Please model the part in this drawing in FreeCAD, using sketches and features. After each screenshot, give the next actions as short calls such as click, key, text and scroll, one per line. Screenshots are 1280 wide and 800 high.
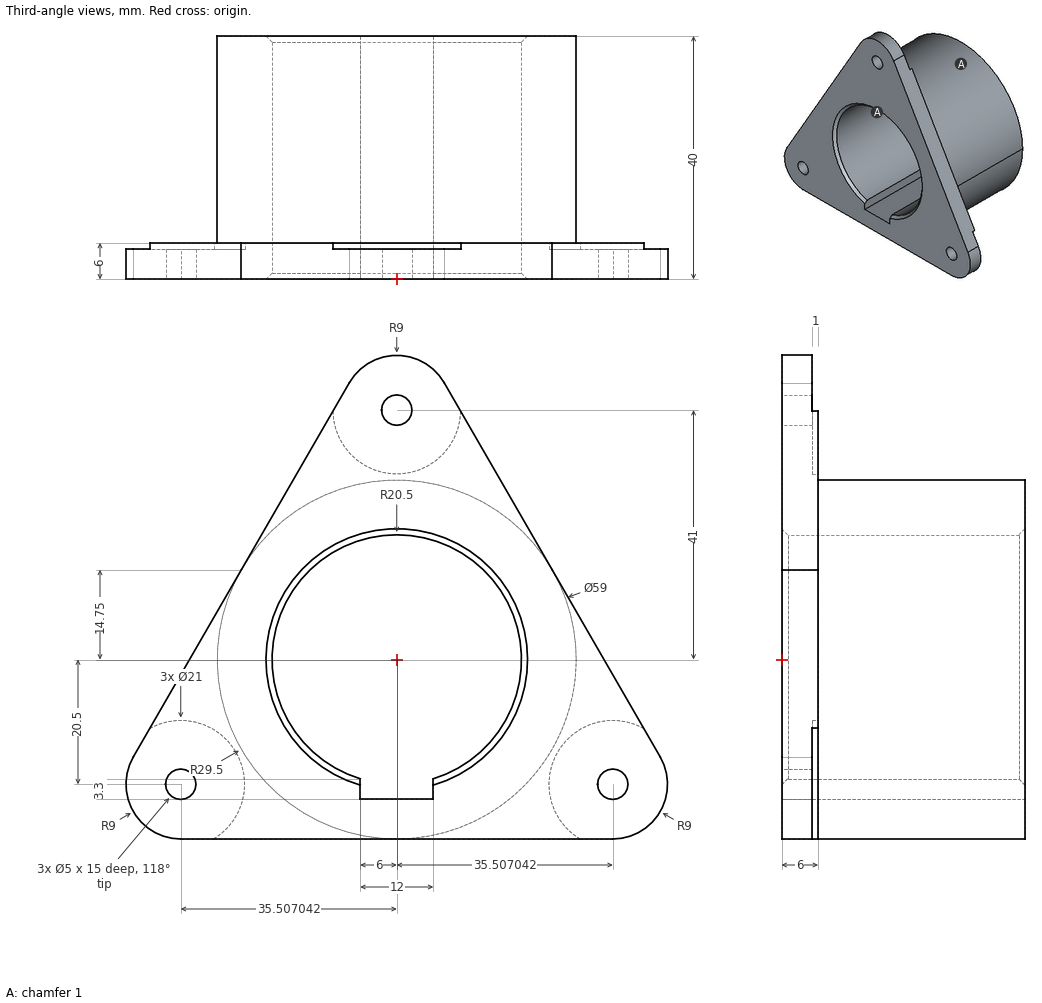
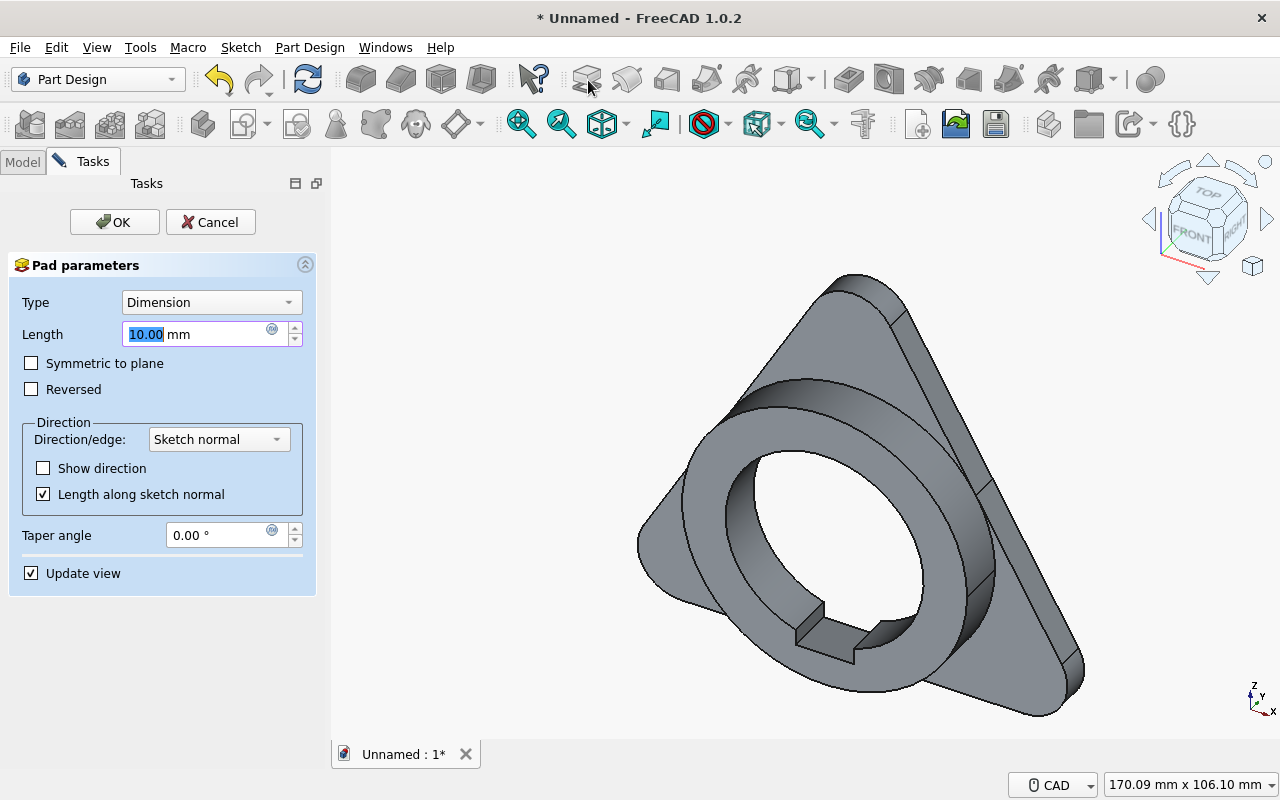
text(40)
key(Tab)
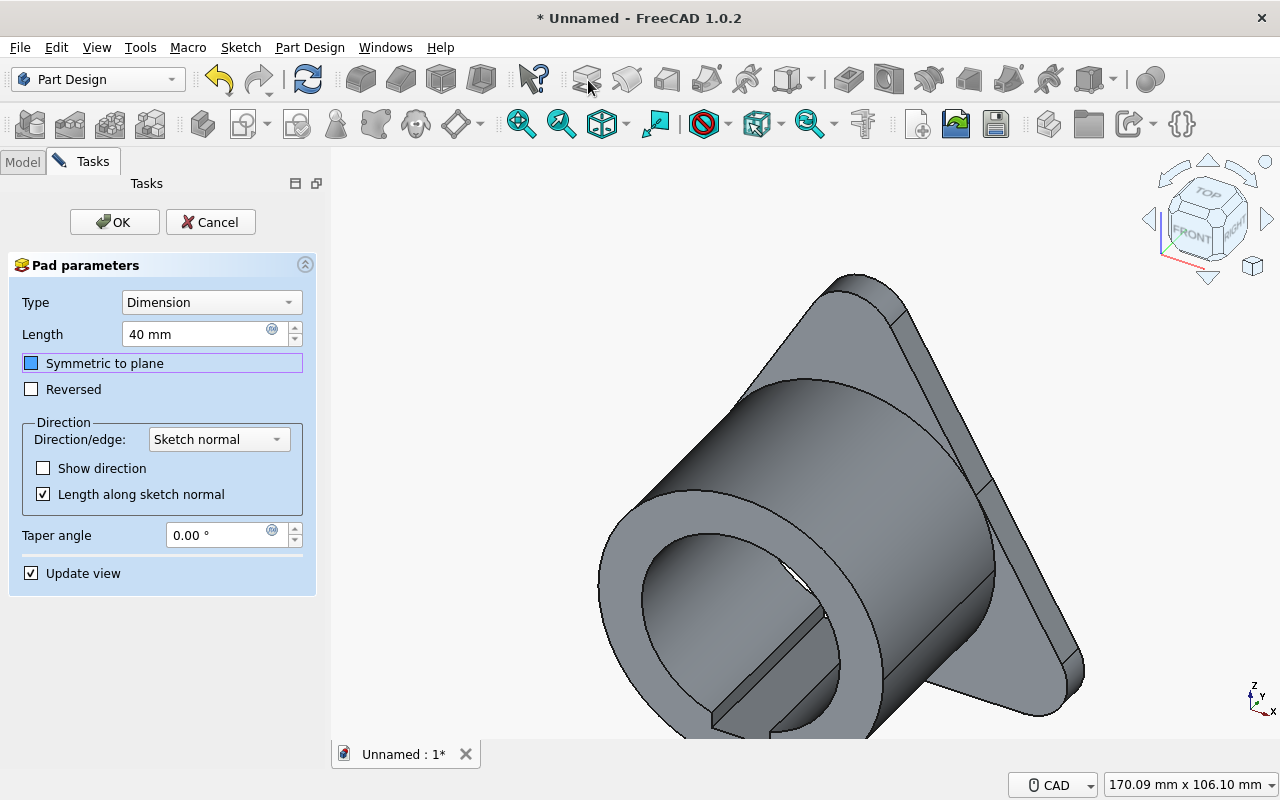
click(30, 389)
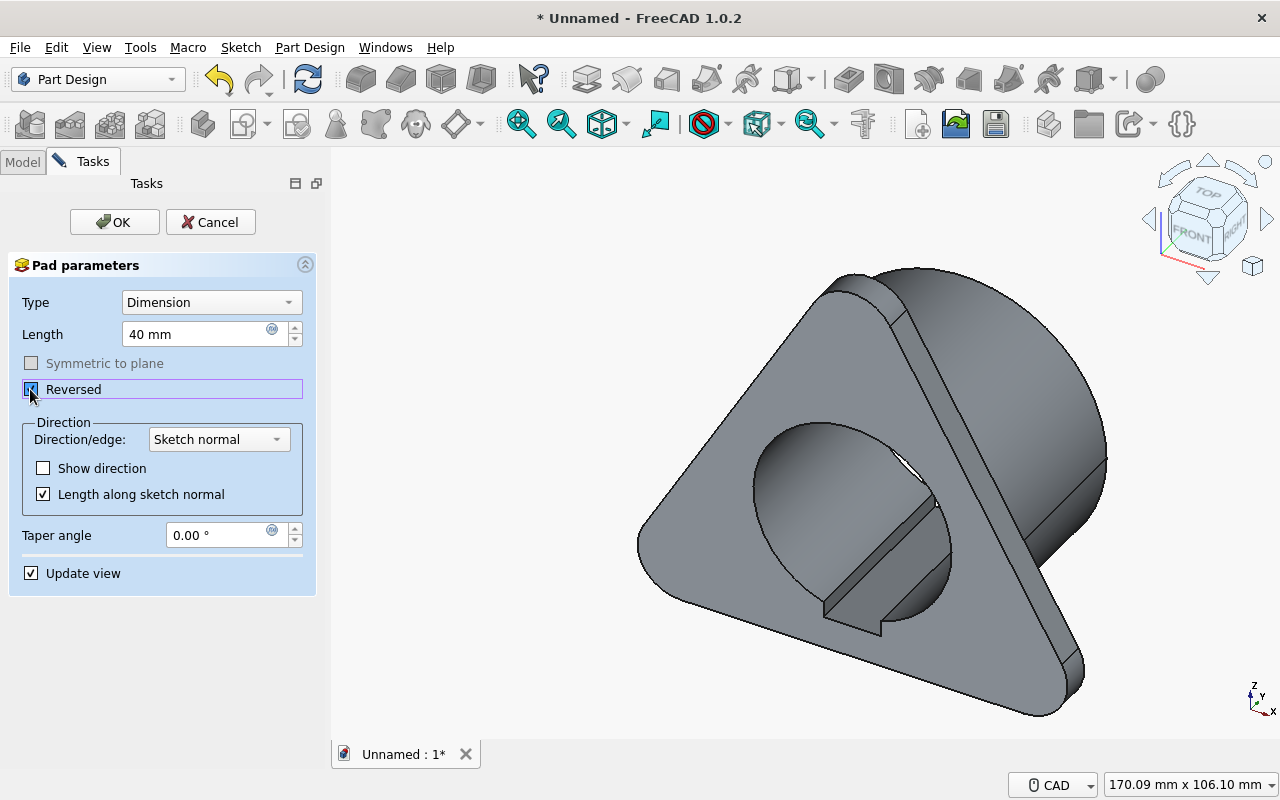
click(115, 222)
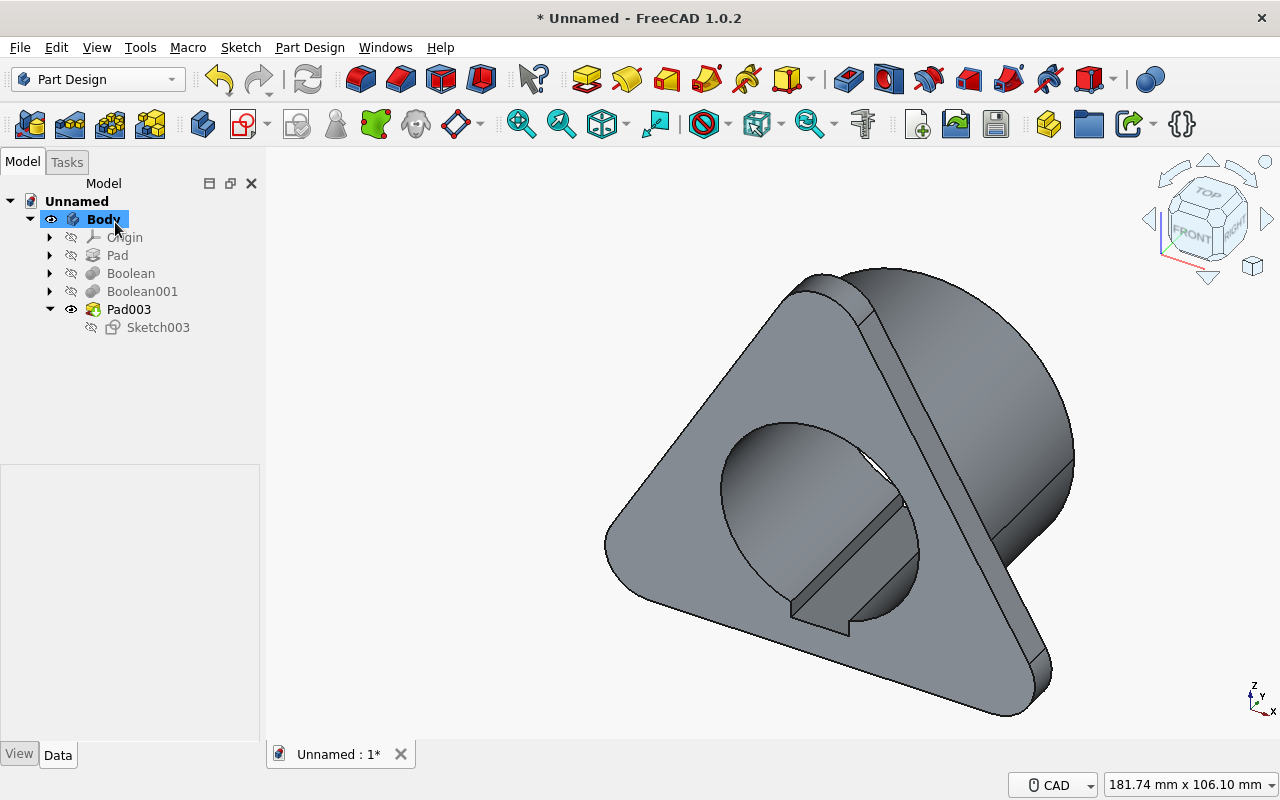
click(522, 124)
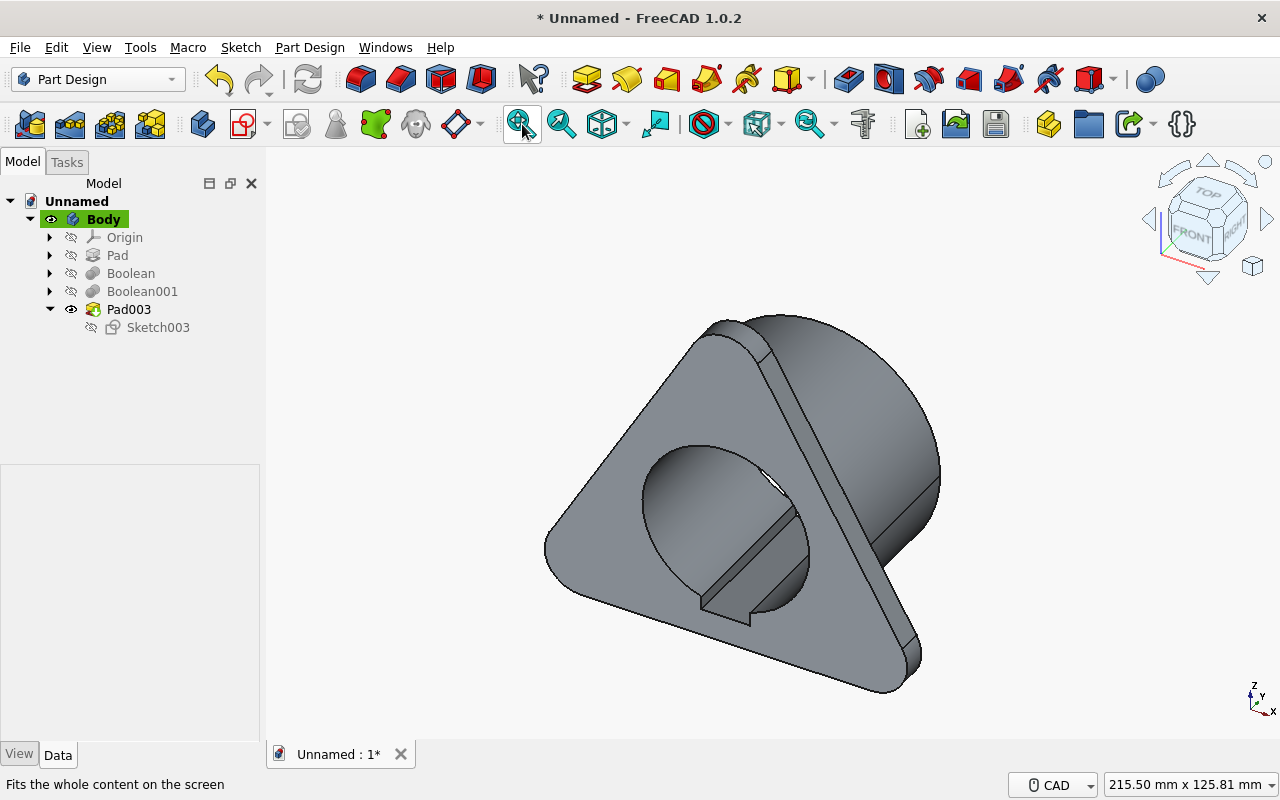
click(650, 470)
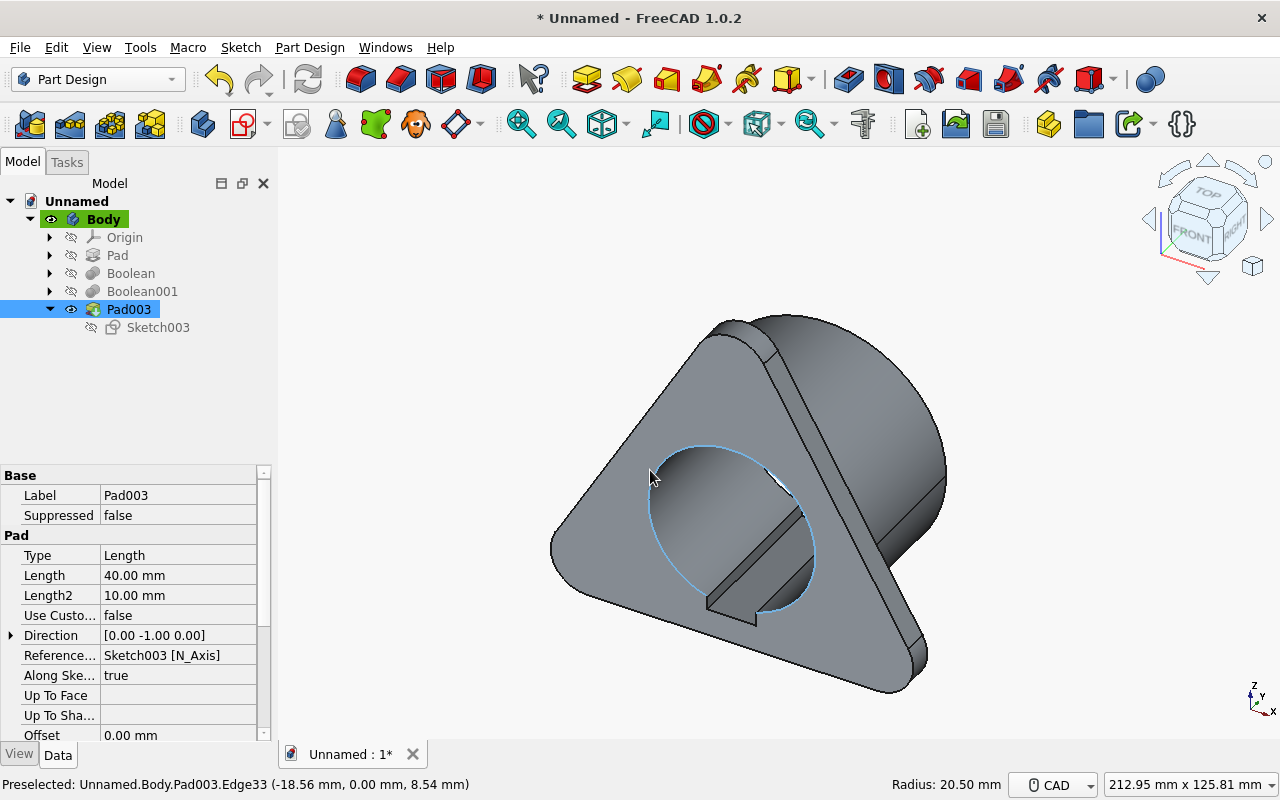
key(0)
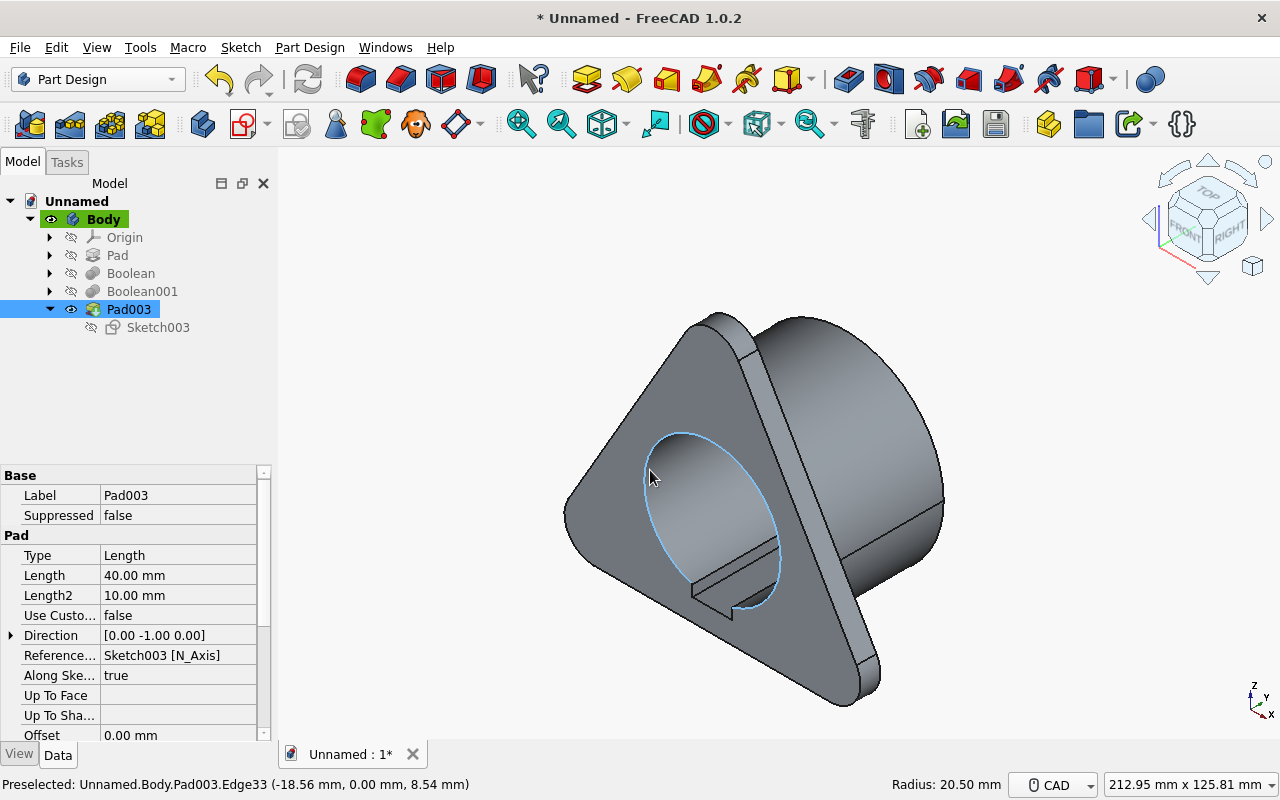
key(2)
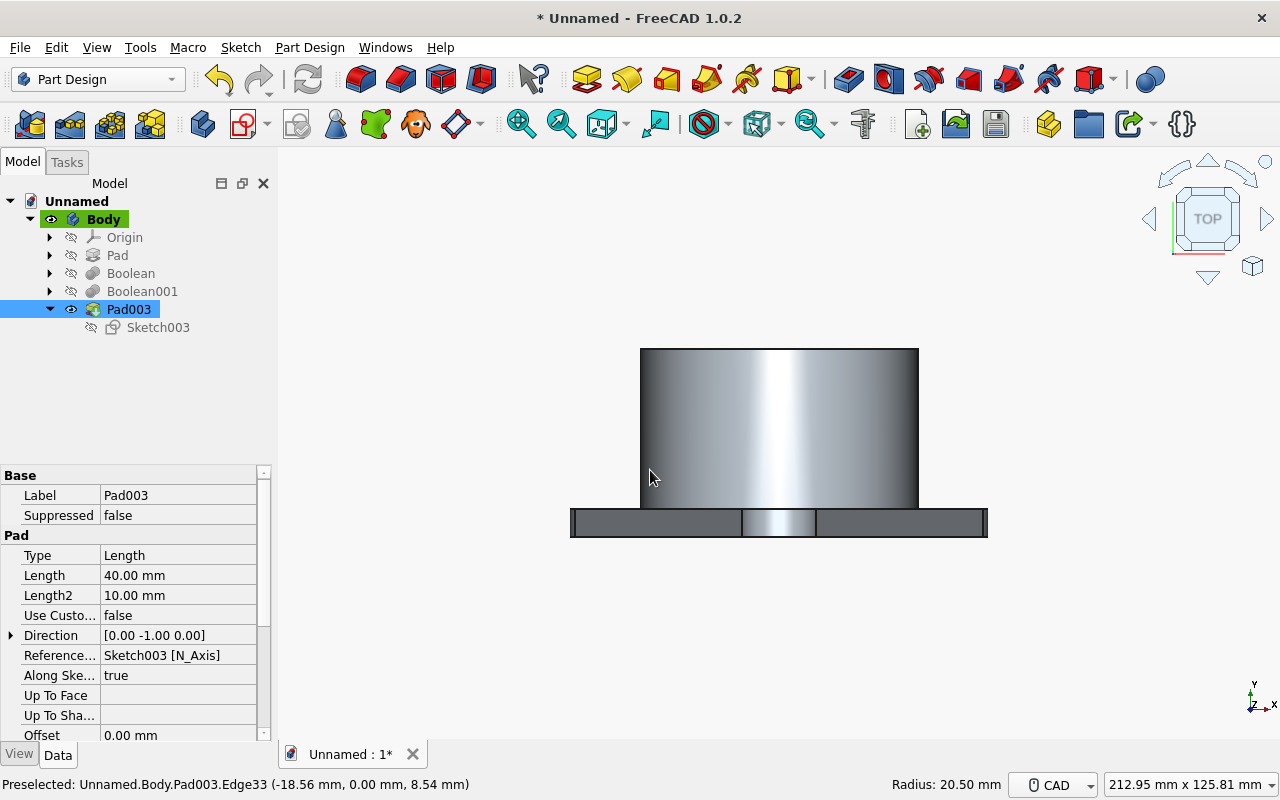
click(522, 124)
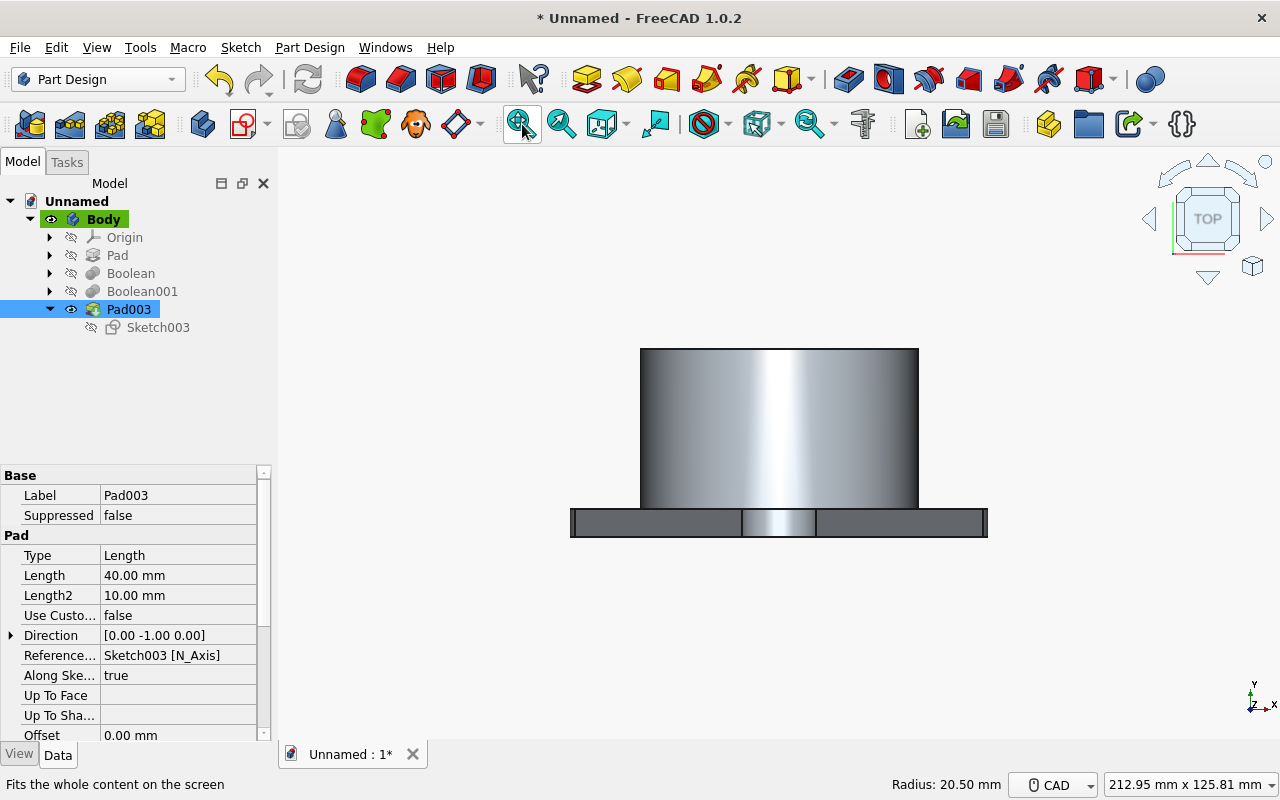
key(1)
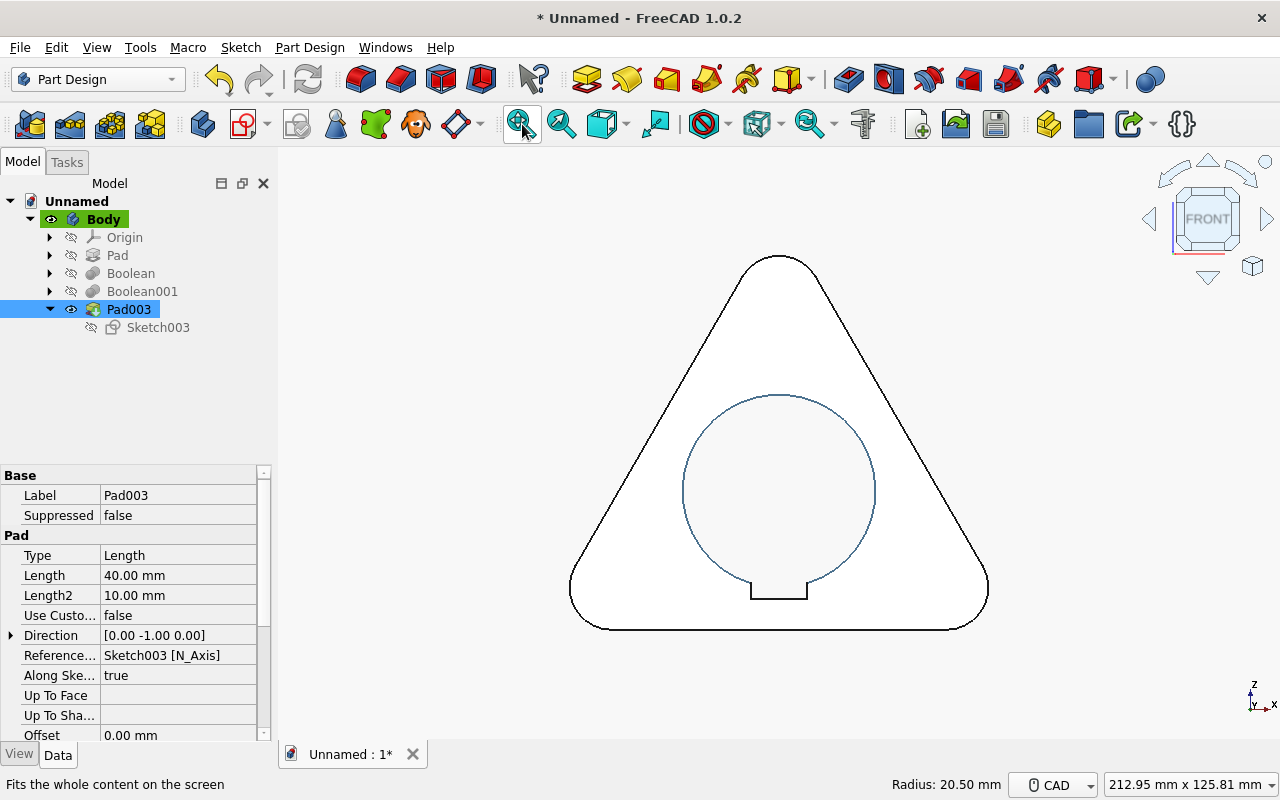
key(3)